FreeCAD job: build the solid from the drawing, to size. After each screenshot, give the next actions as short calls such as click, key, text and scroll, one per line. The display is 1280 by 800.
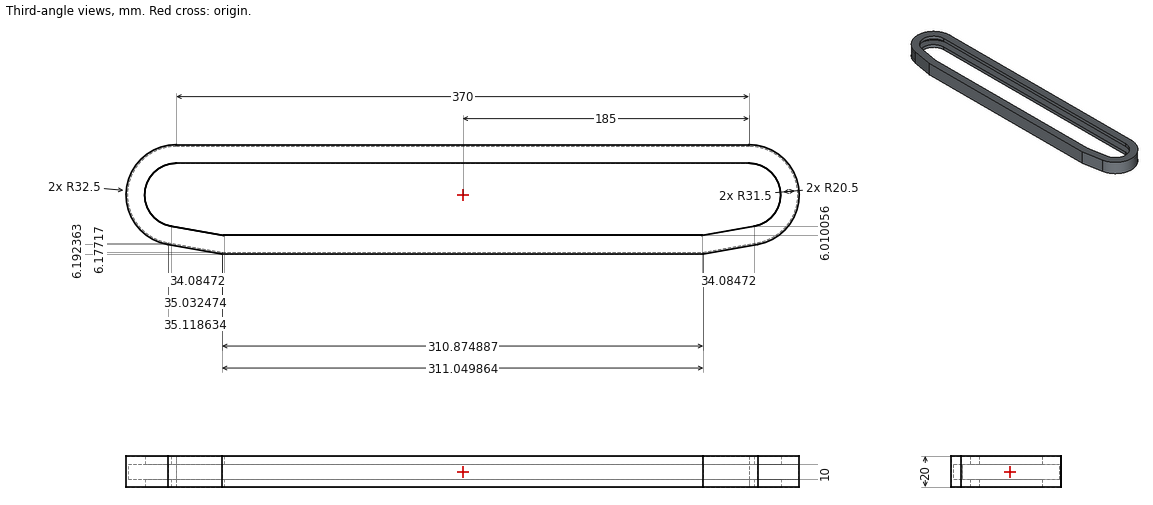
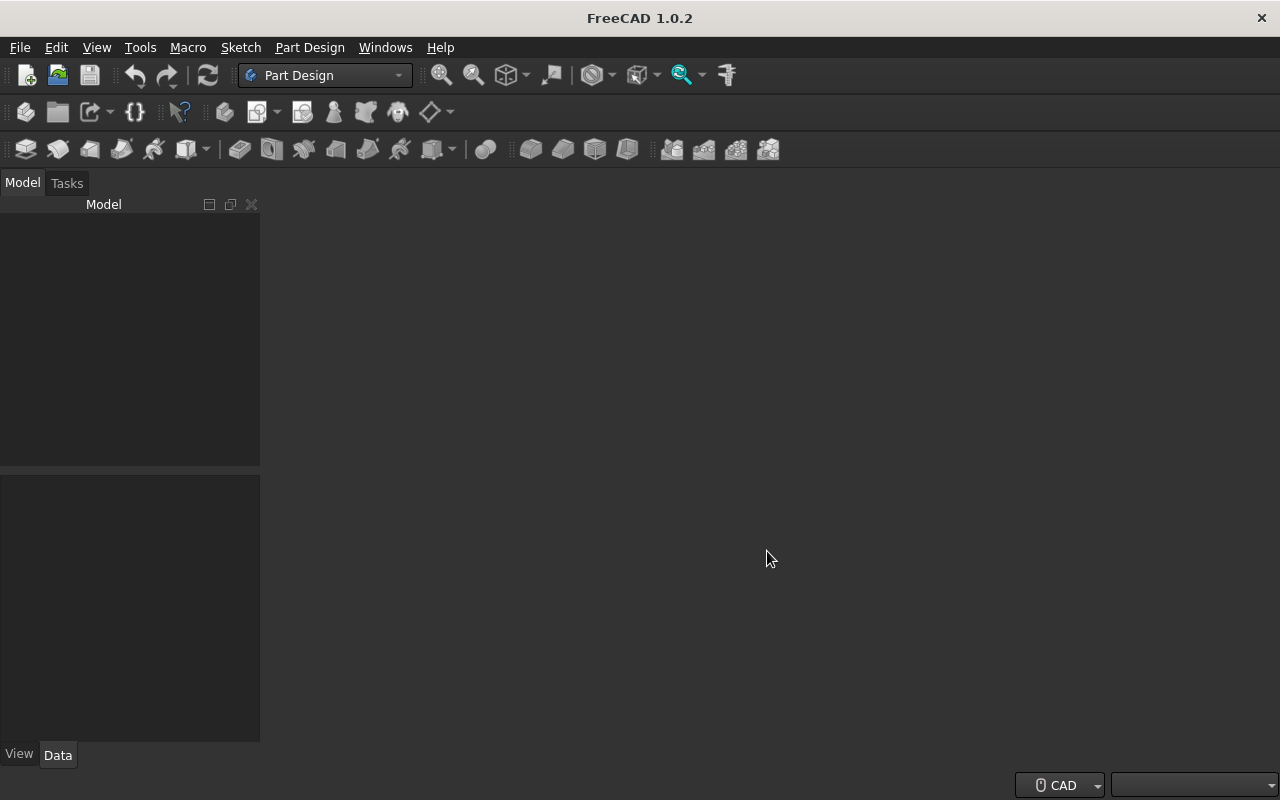
key(ctrl+n)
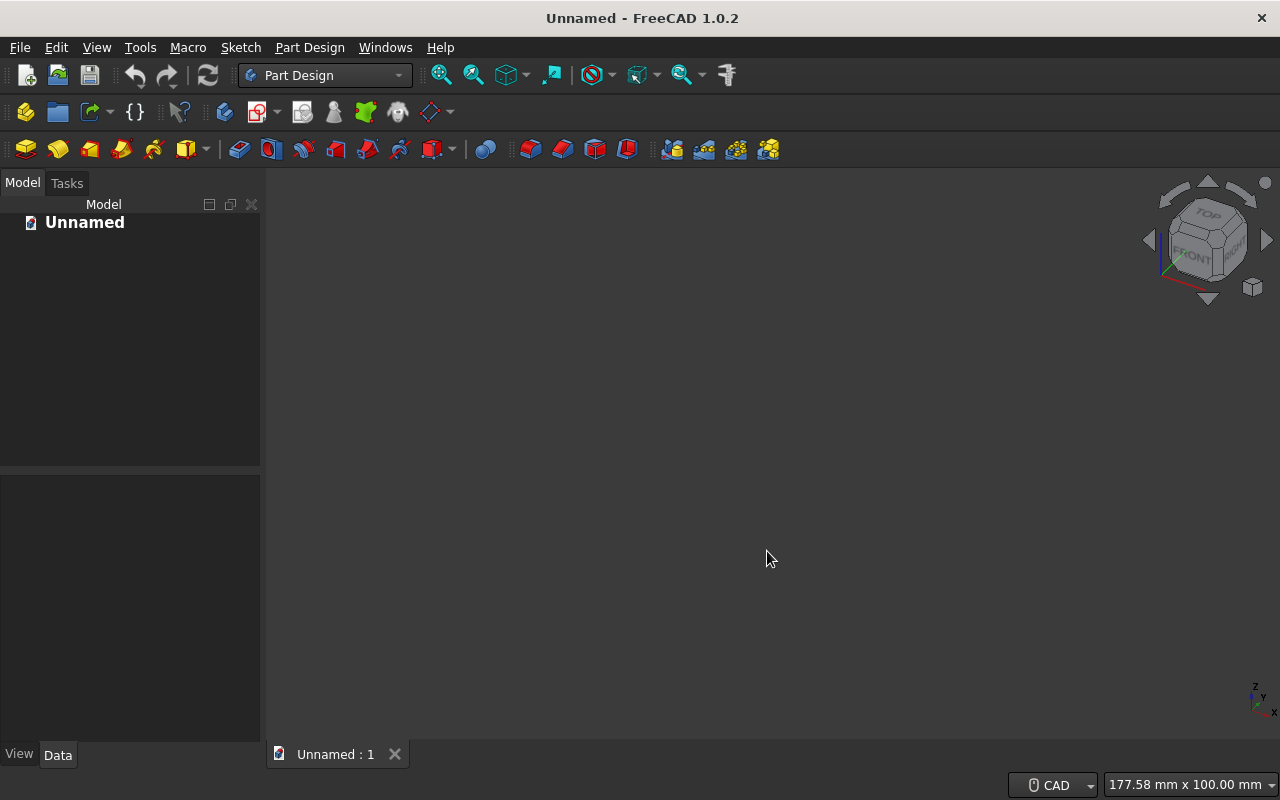
click(258, 112)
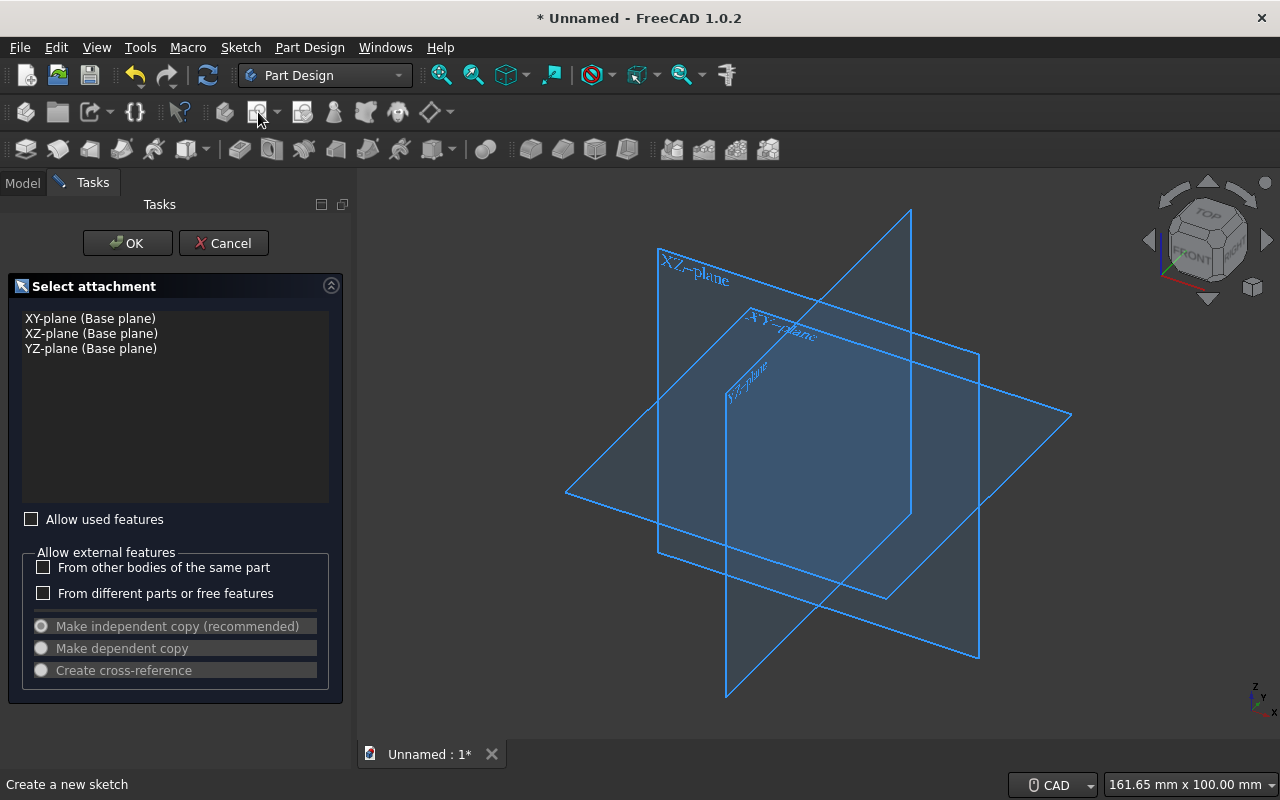
click(82, 318)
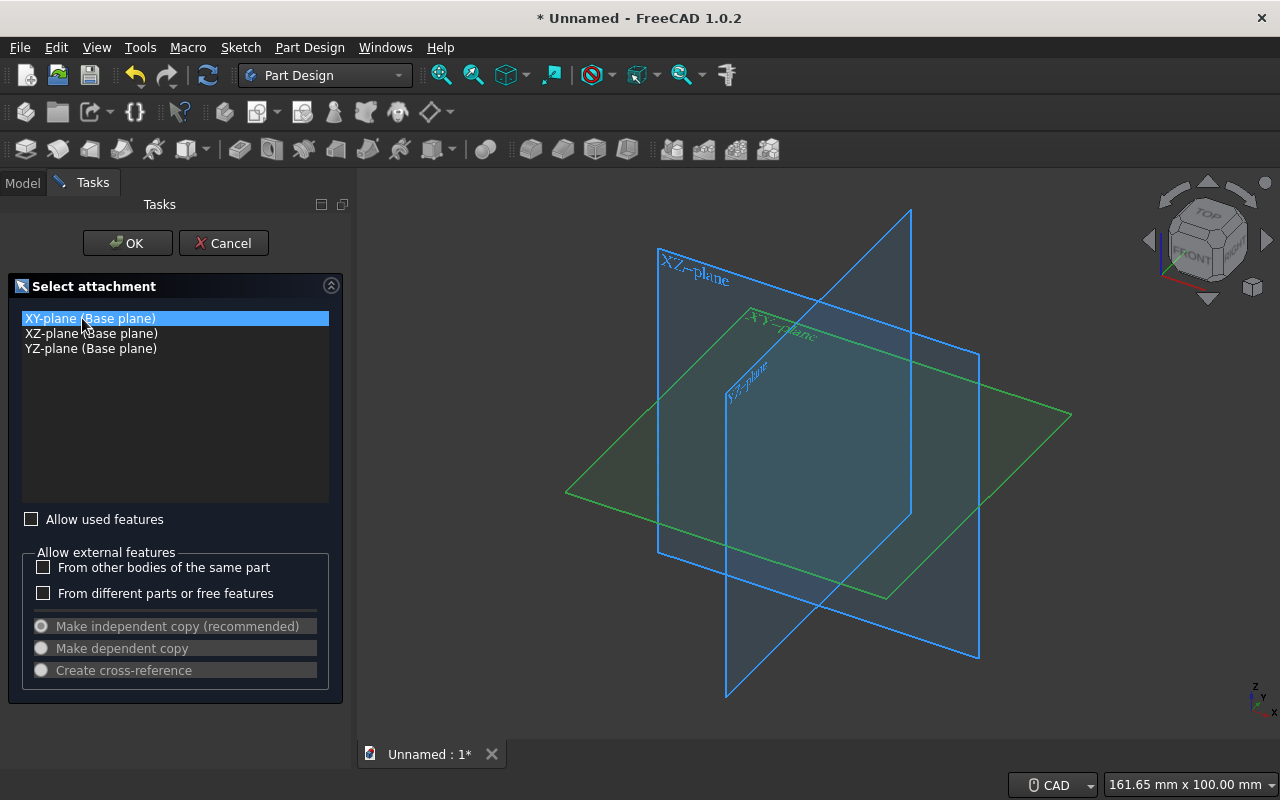
click(128, 243)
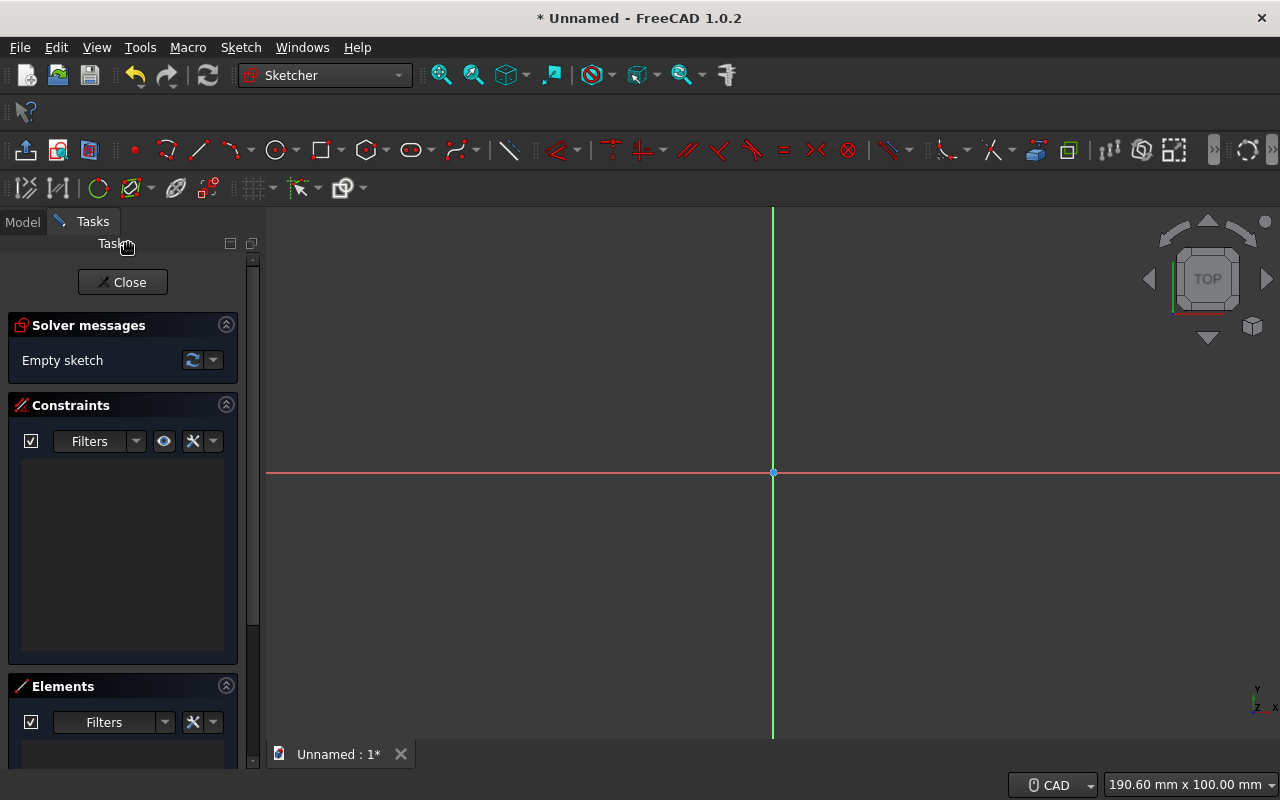
scroll(682, 468, down, 7)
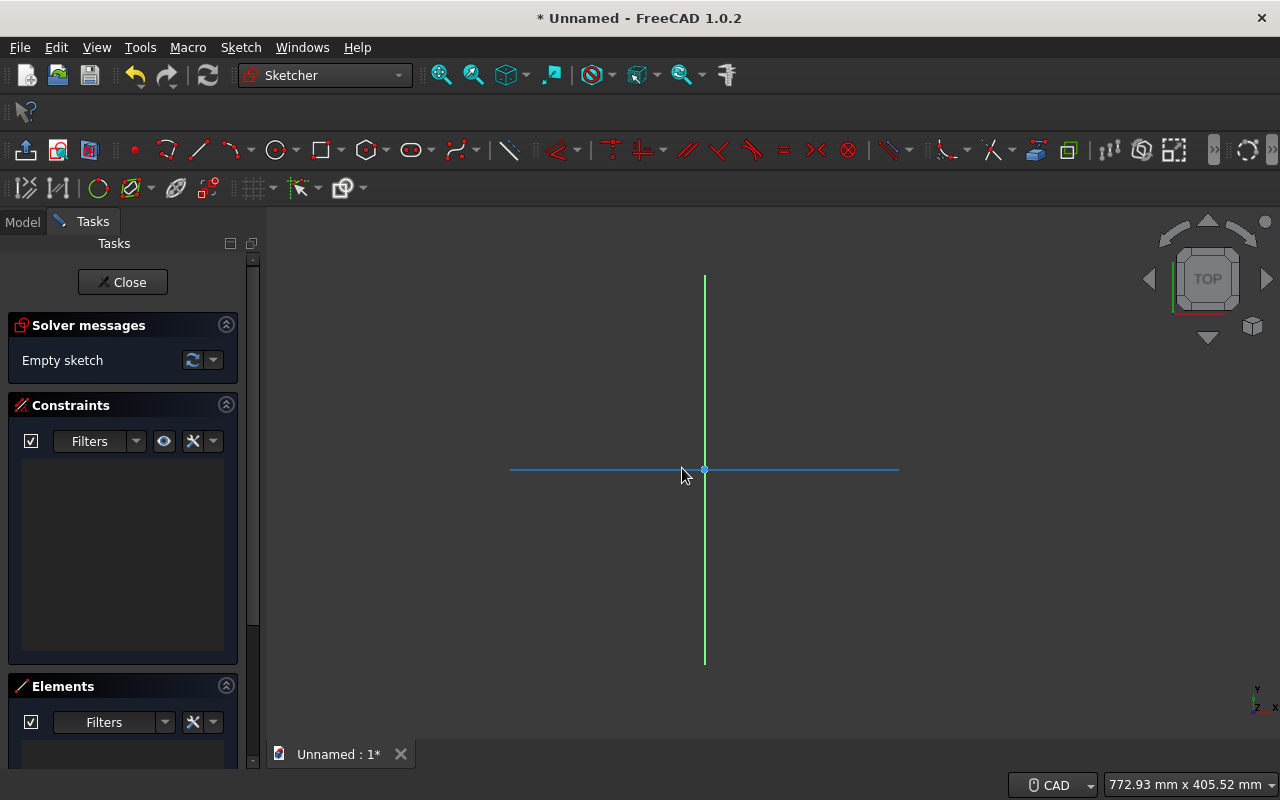
key(g)
key(l)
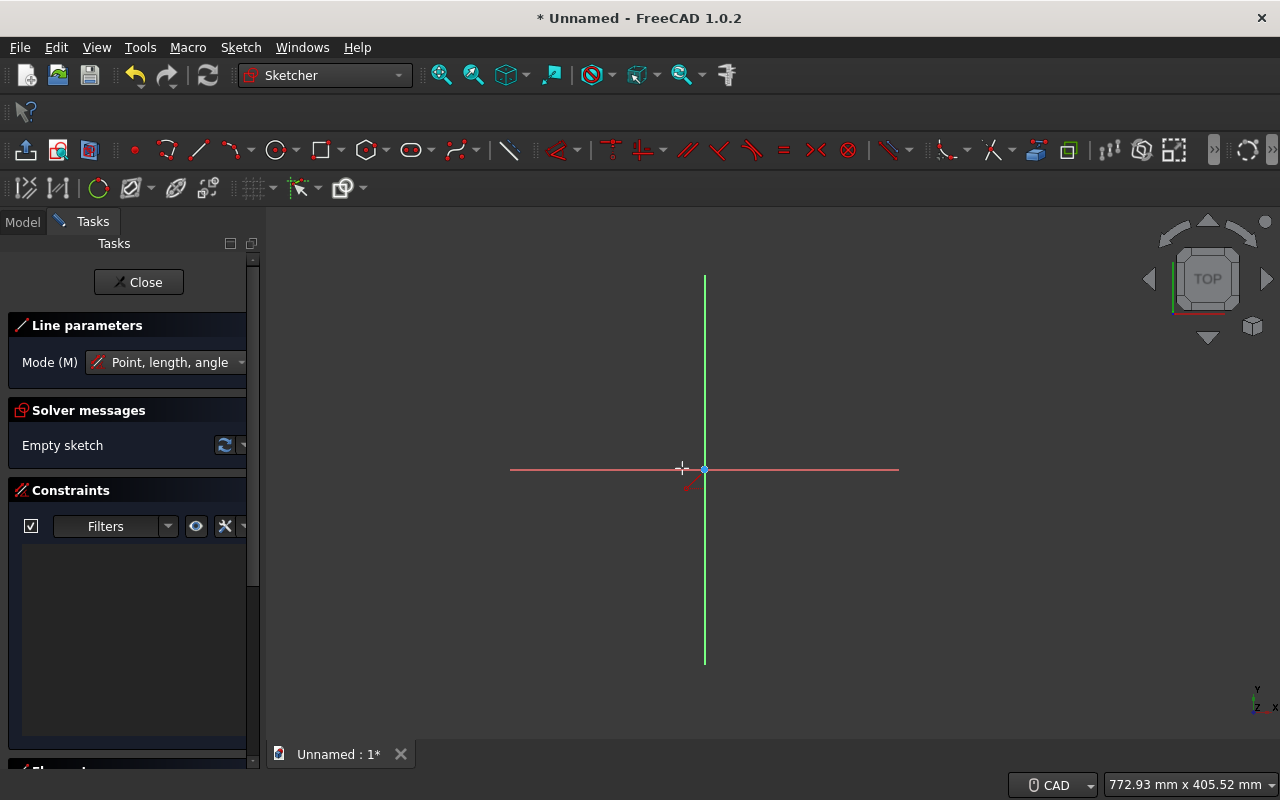
click(947, 427)
click(462, 427)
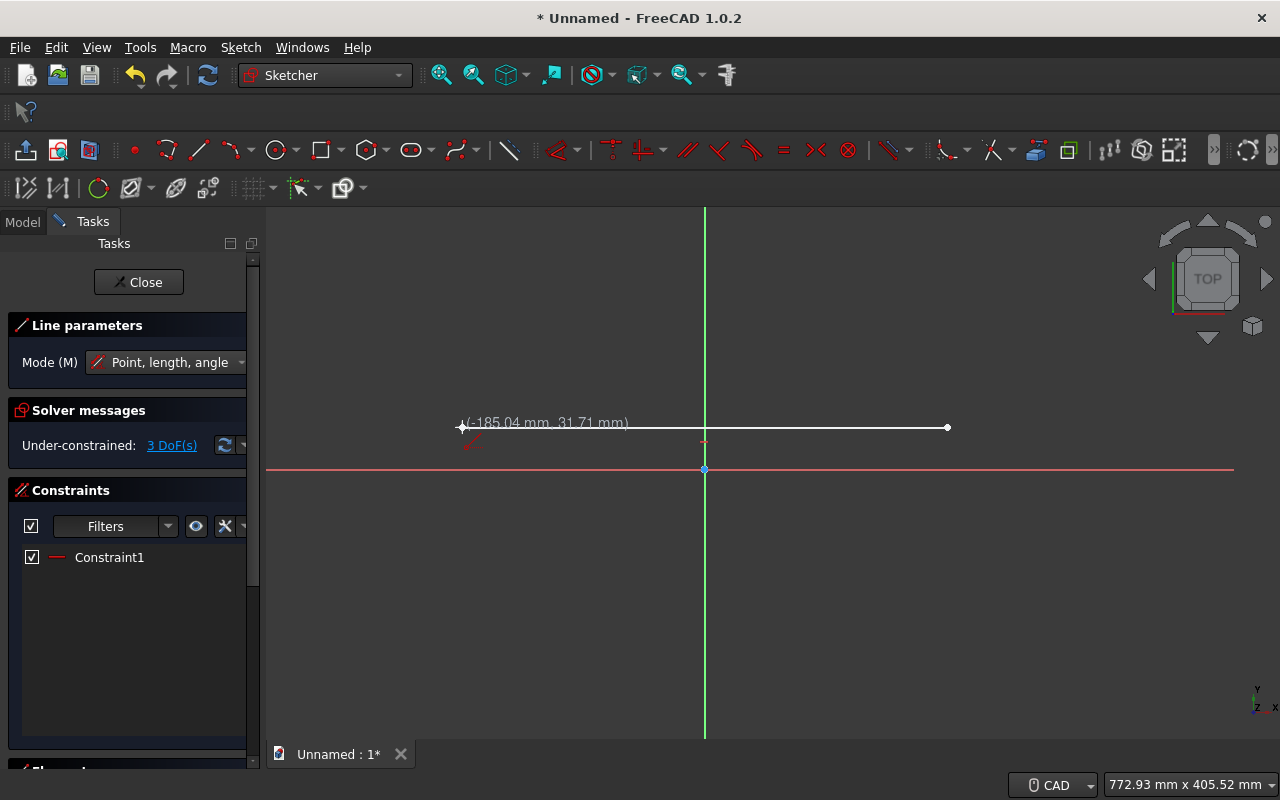
key(g)
key(m)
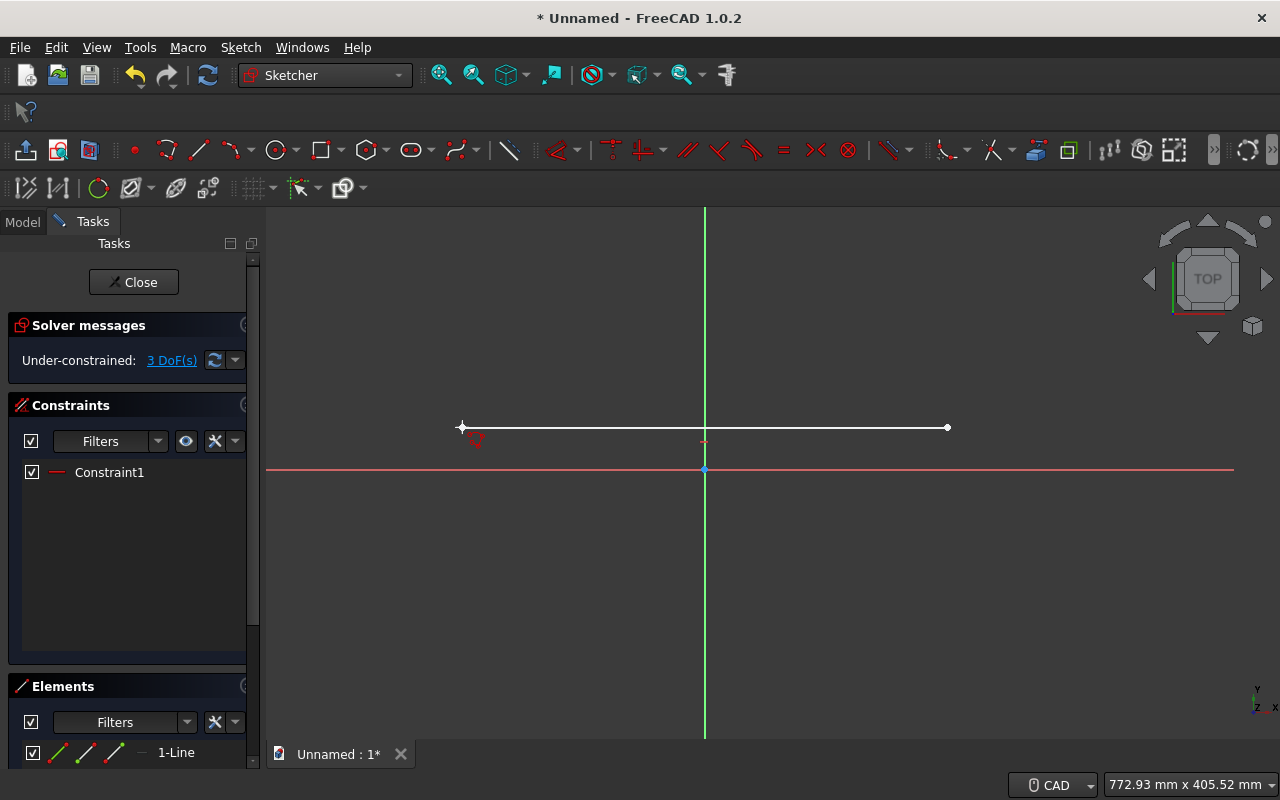
click(455, 512)
click(501, 520)
click(909, 520)
click(955, 512)
right_click(955, 512)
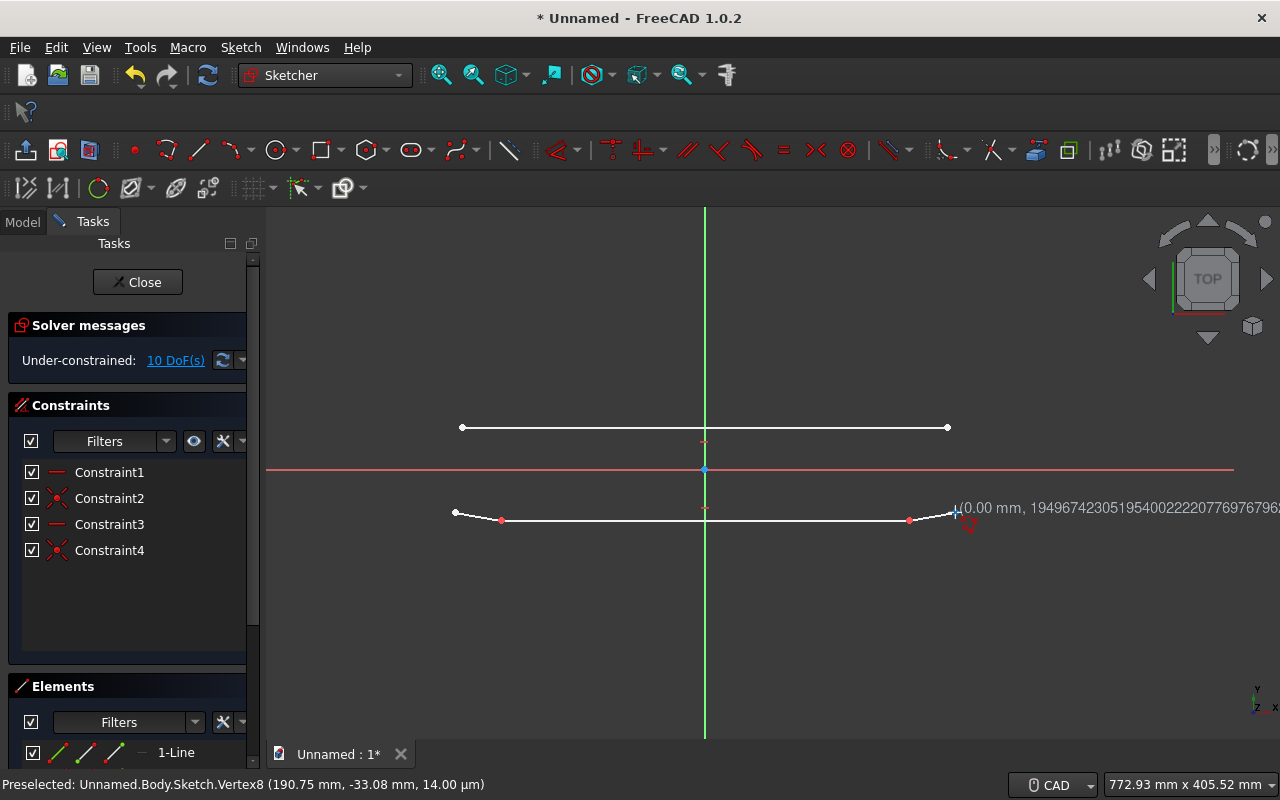
click(232, 150)